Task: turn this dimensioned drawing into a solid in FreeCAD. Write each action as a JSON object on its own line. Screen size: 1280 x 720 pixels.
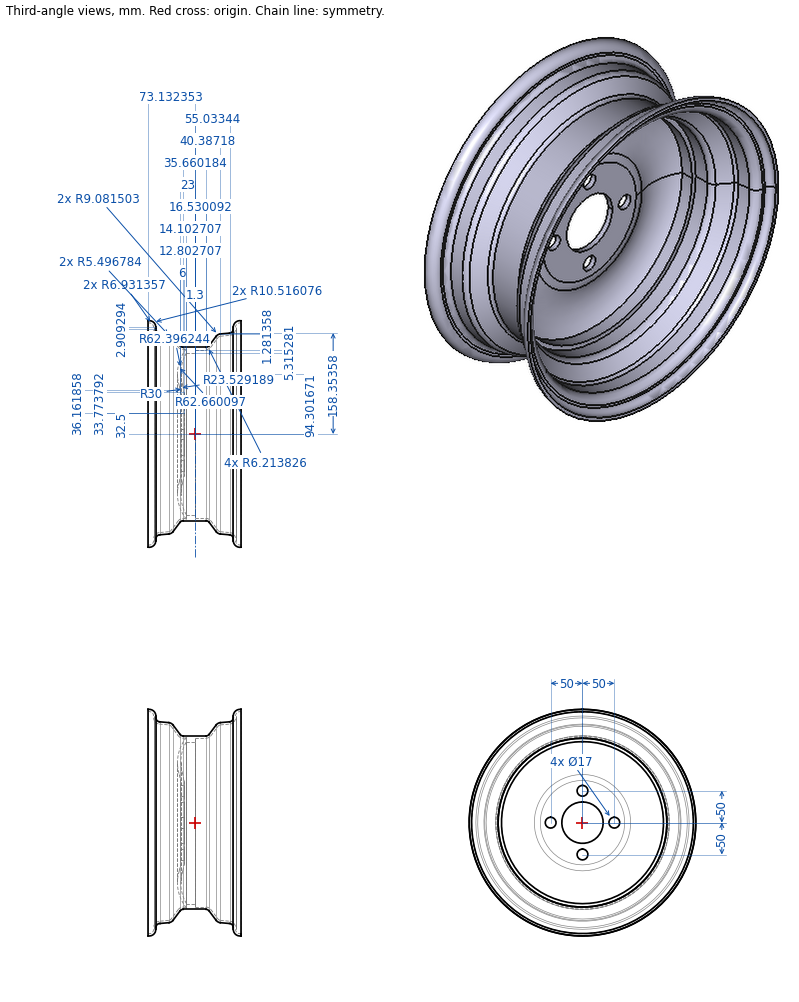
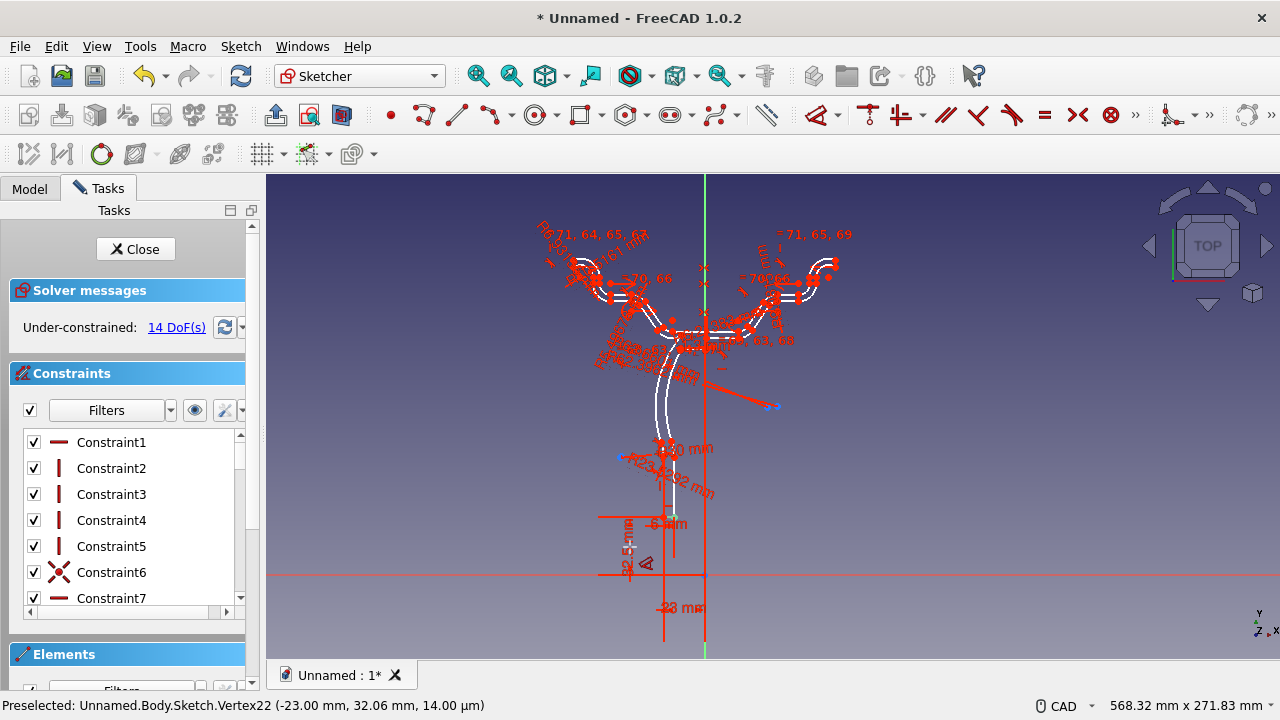
{"action": "scroll", "coordinate": [600, 281], "scroll_direction": "up", "scroll_amount": 11}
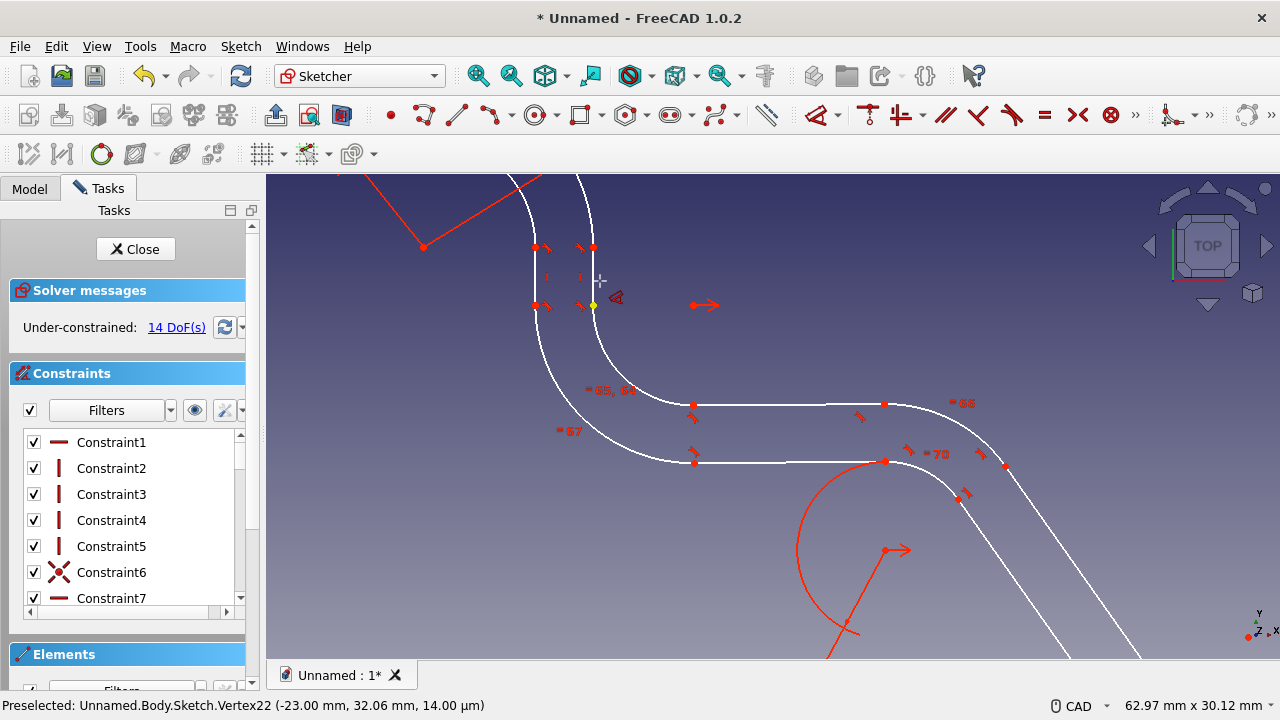
{"action": "left_click", "coordinate": [593, 276]}
{"action": "left_click", "coordinate": [559, 276]}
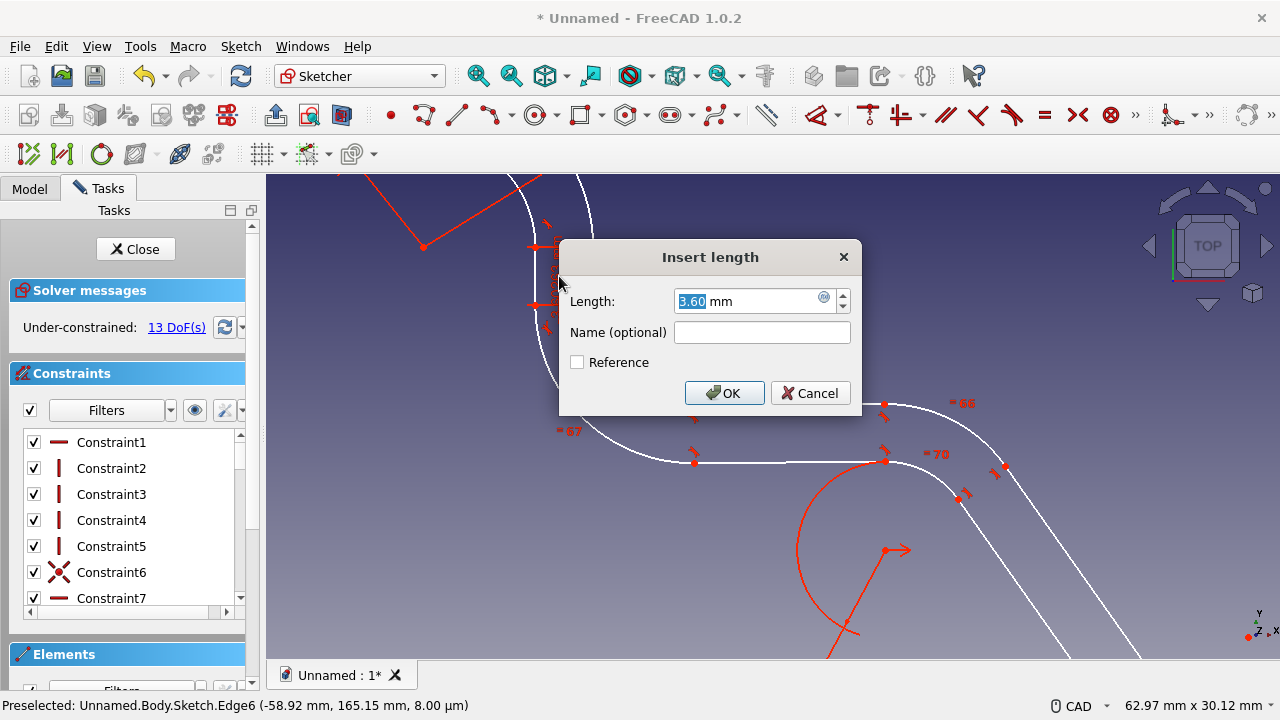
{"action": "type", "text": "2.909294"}
{"action": "key", "text": "Return"}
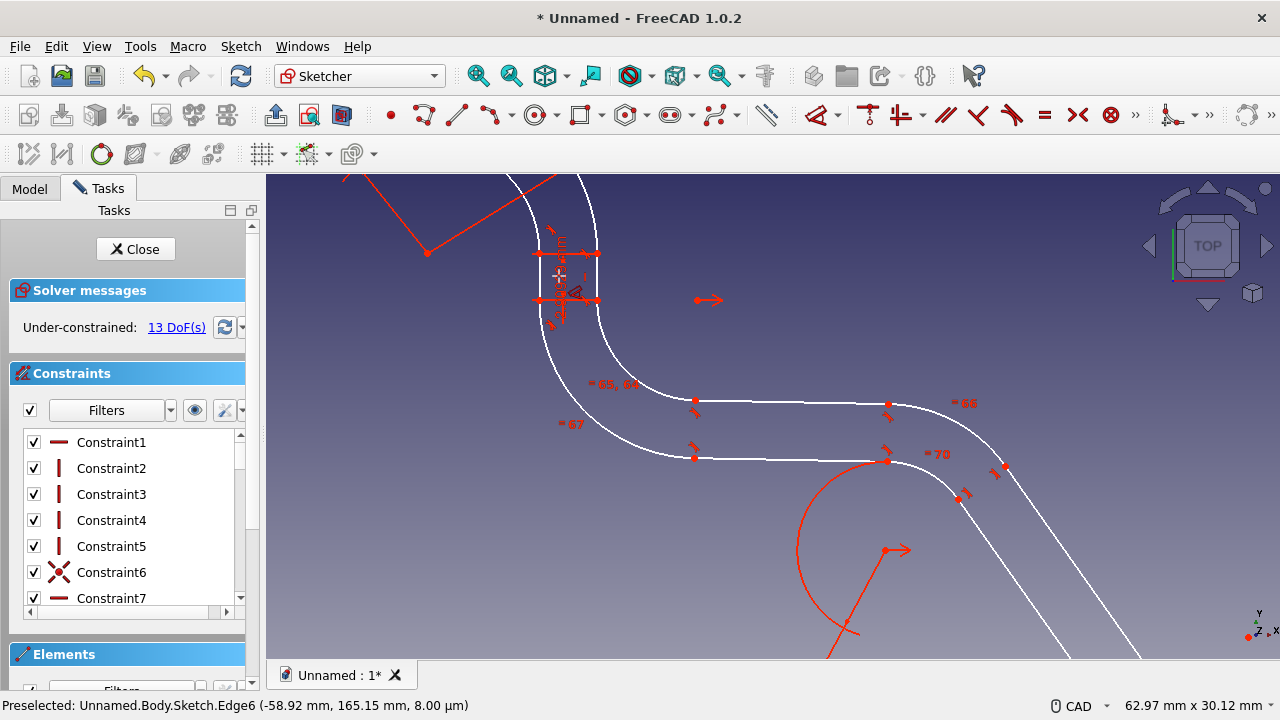
{"action": "scroll", "coordinate": [600, 281], "scroll_direction": "down", "scroll_amount": 11}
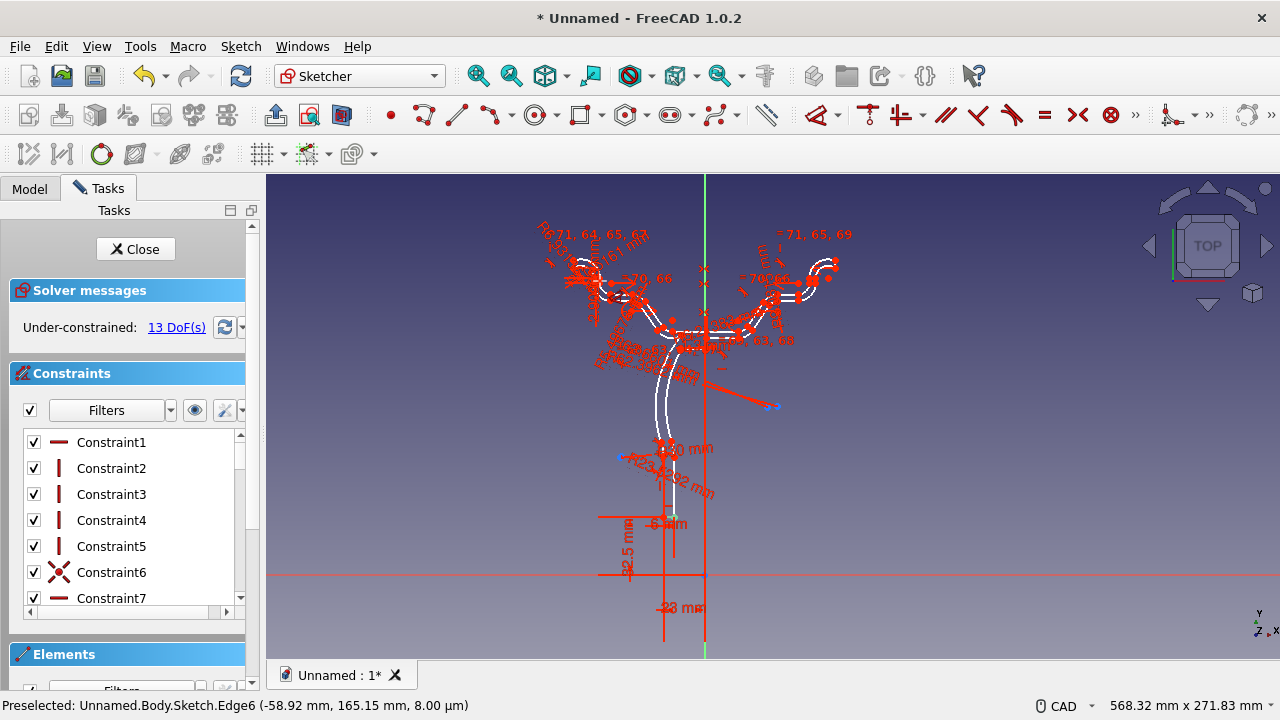
{"action": "scroll", "coordinate": [707, 346], "scroll_direction": "up", "scroll_amount": 9}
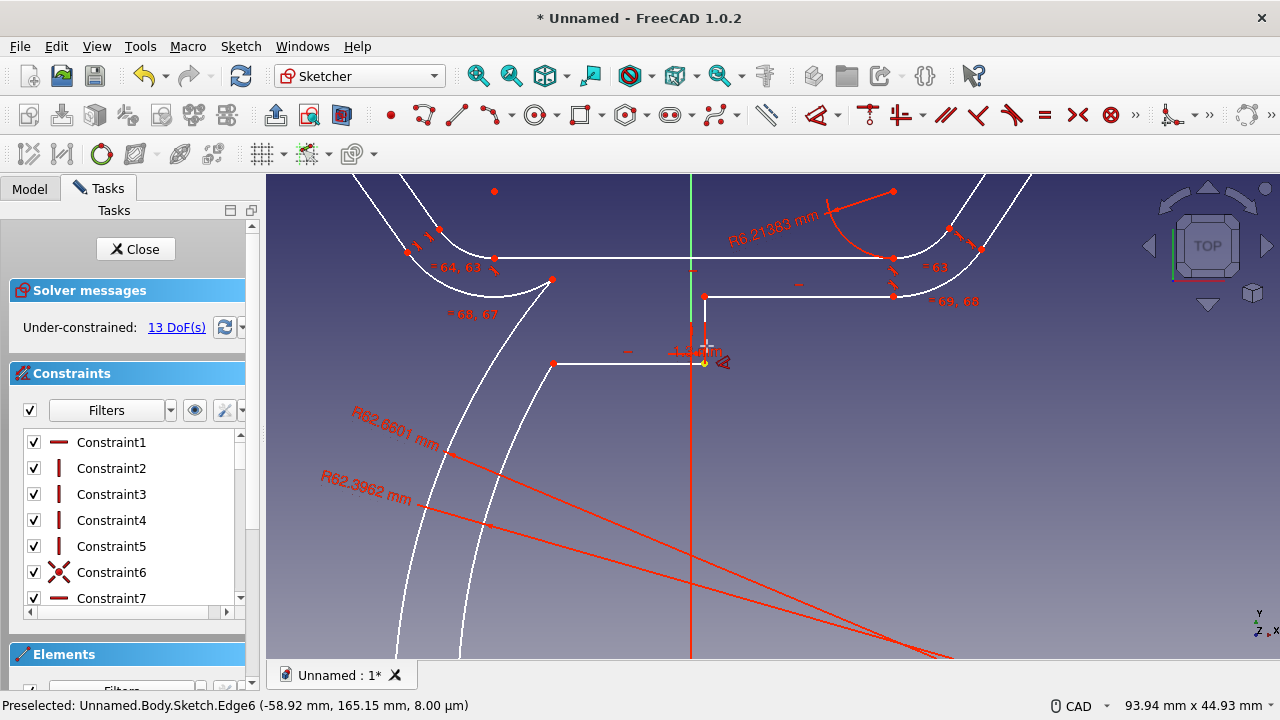
{"action": "left_click", "coordinate": [705, 344]}
{"action": "left_click", "coordinate": [739, 330]}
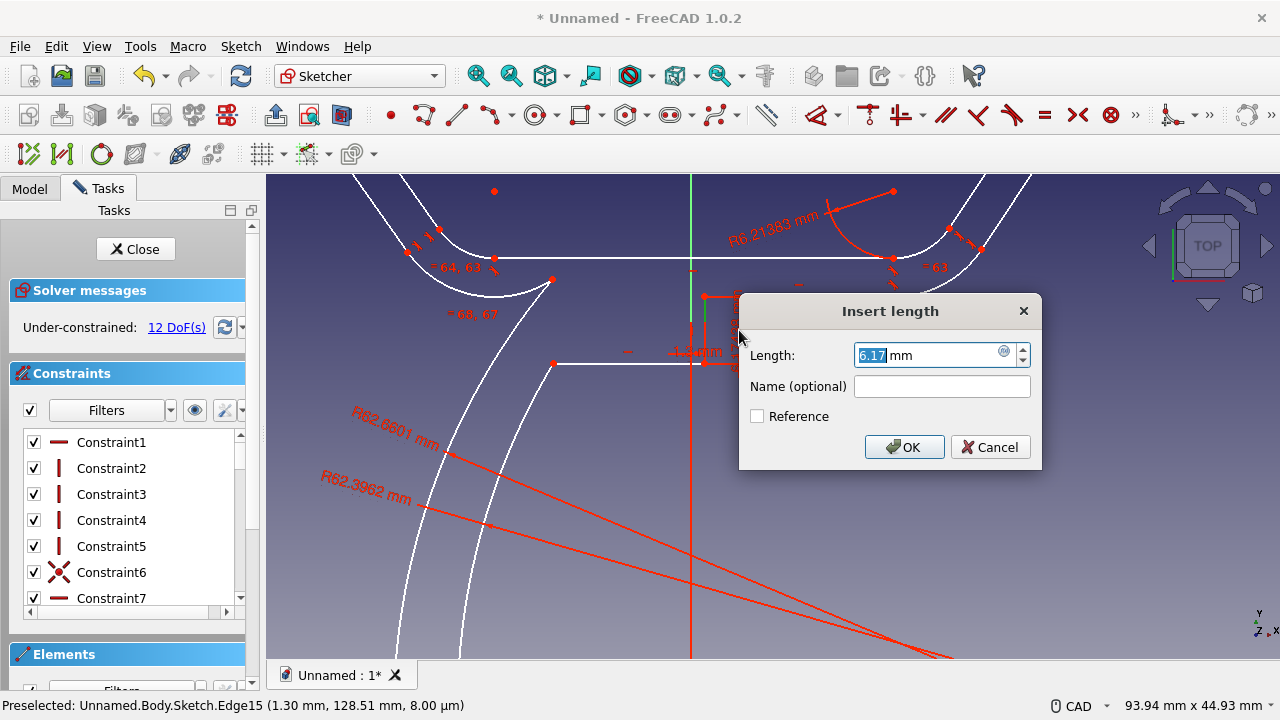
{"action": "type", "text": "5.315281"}
{"action": "key", "text": "Return"}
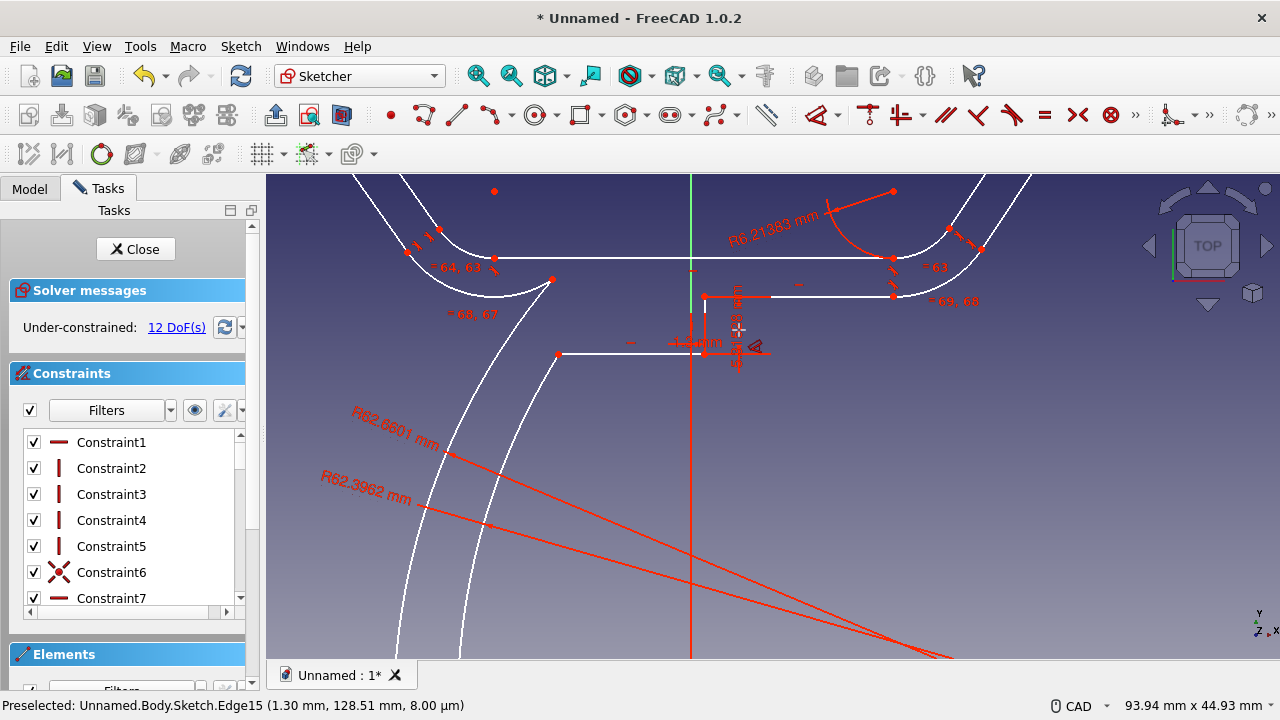
{"action": "left_click", "coordinate": [774, 258]}
{"action": "left_click", "coordinate": [602, 224]}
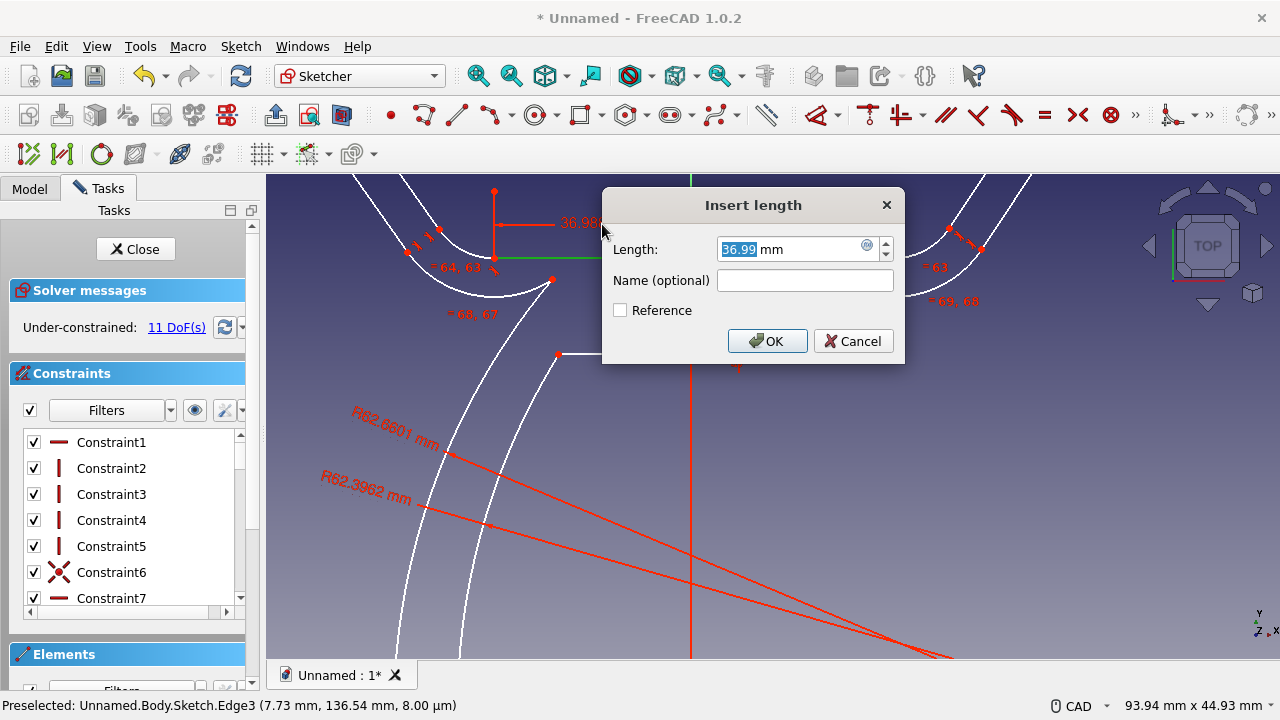
{"action": "type", "text": "35.660184"}
{"action": "key", "text": "Return"}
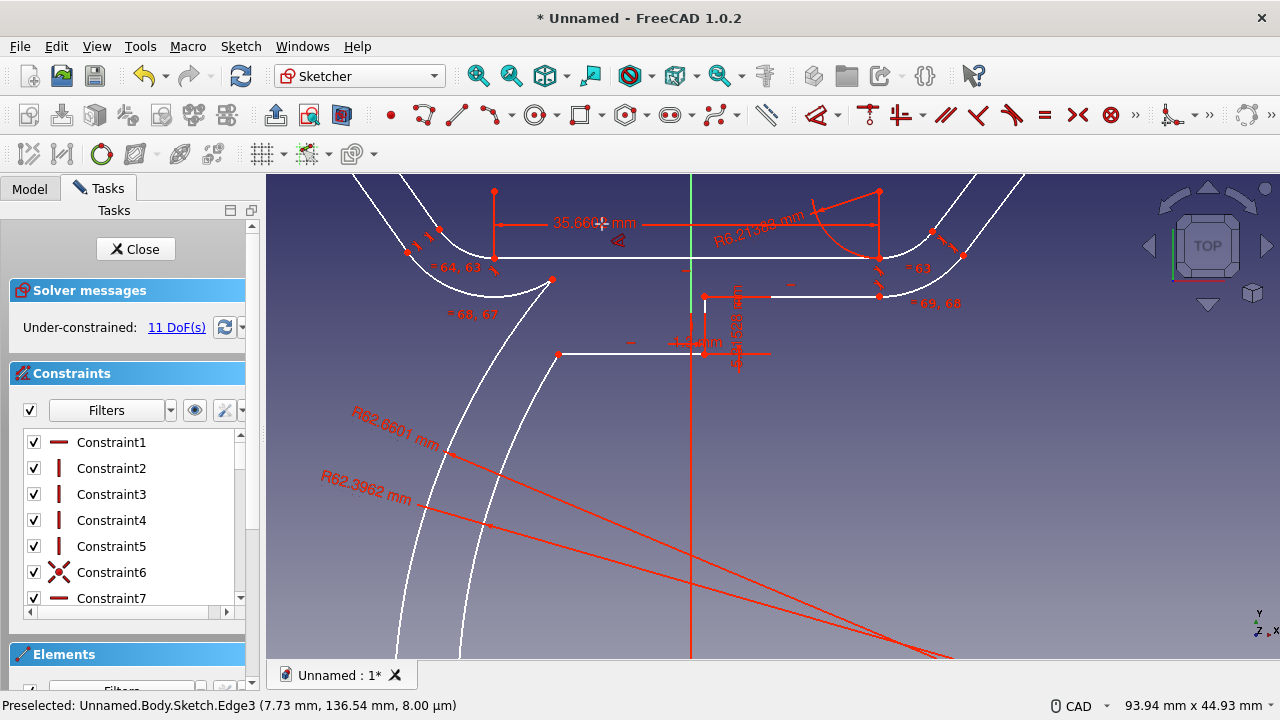
{"action": "scroll", "coordinate": [707, 346], "scroll_direction": "down", "scroll_amount": 9}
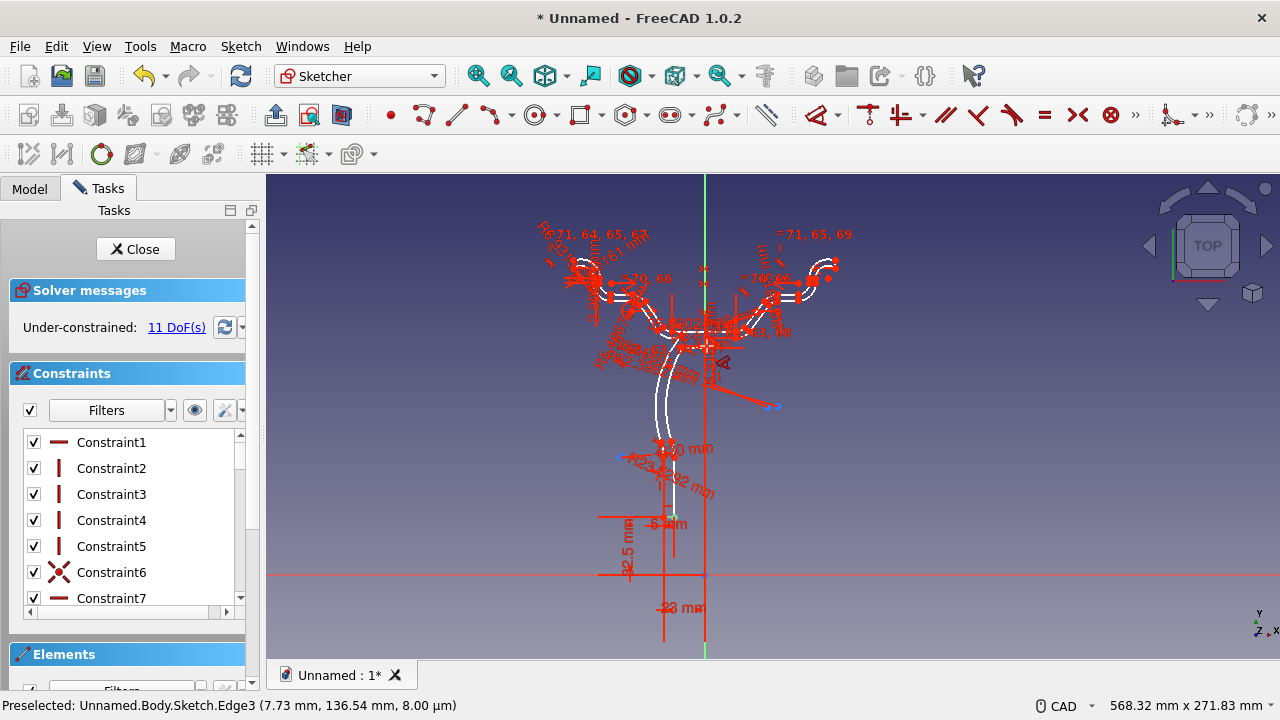
{"action": "scroll", "coordinate": [664, 475], "scroll_direction": "up", "scroll_amount": 2}